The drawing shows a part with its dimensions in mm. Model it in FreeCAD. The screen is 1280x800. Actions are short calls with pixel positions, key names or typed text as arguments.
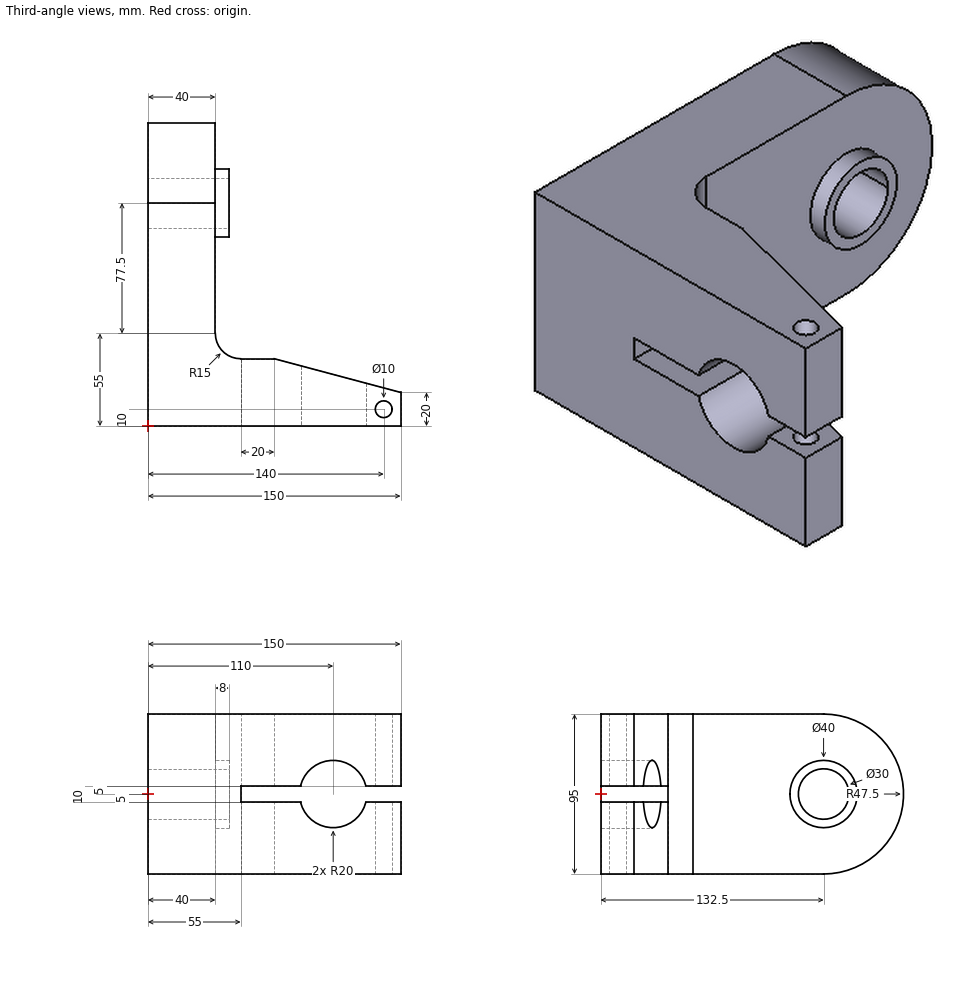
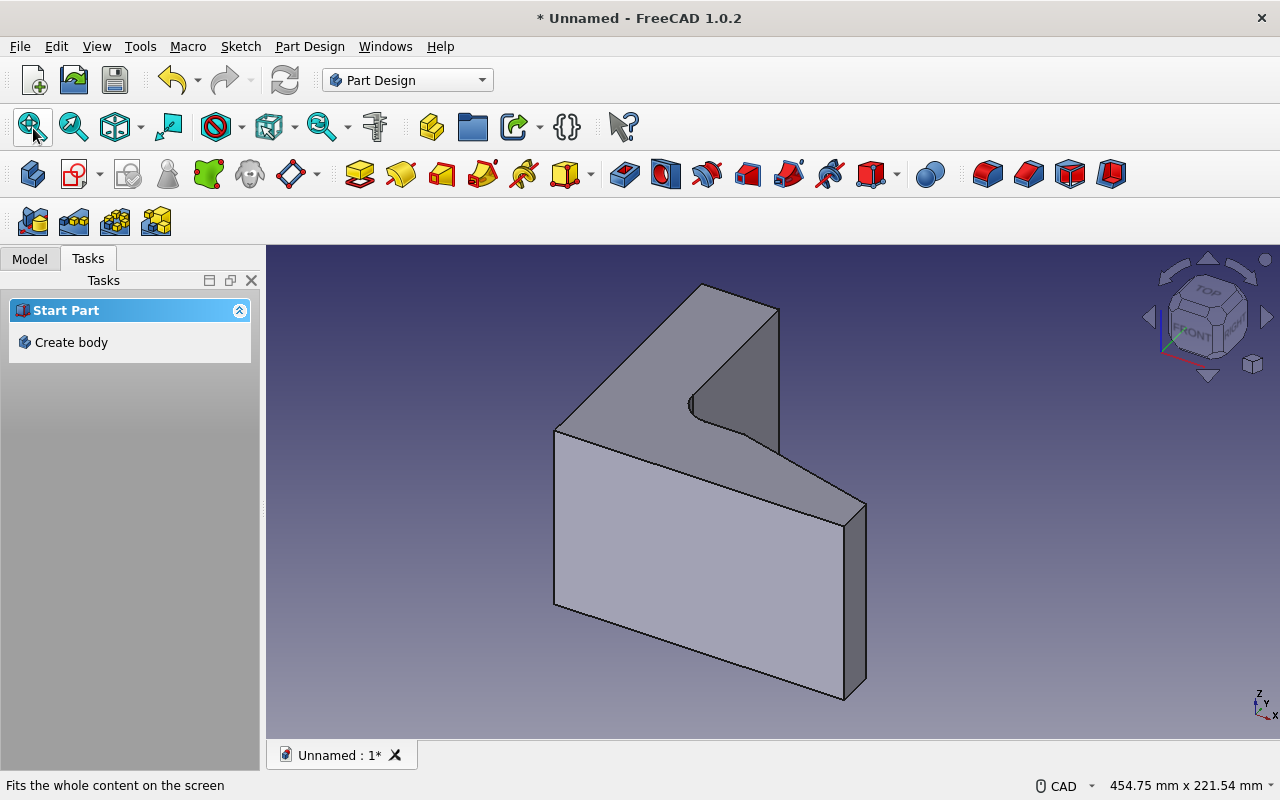
click(74, 174)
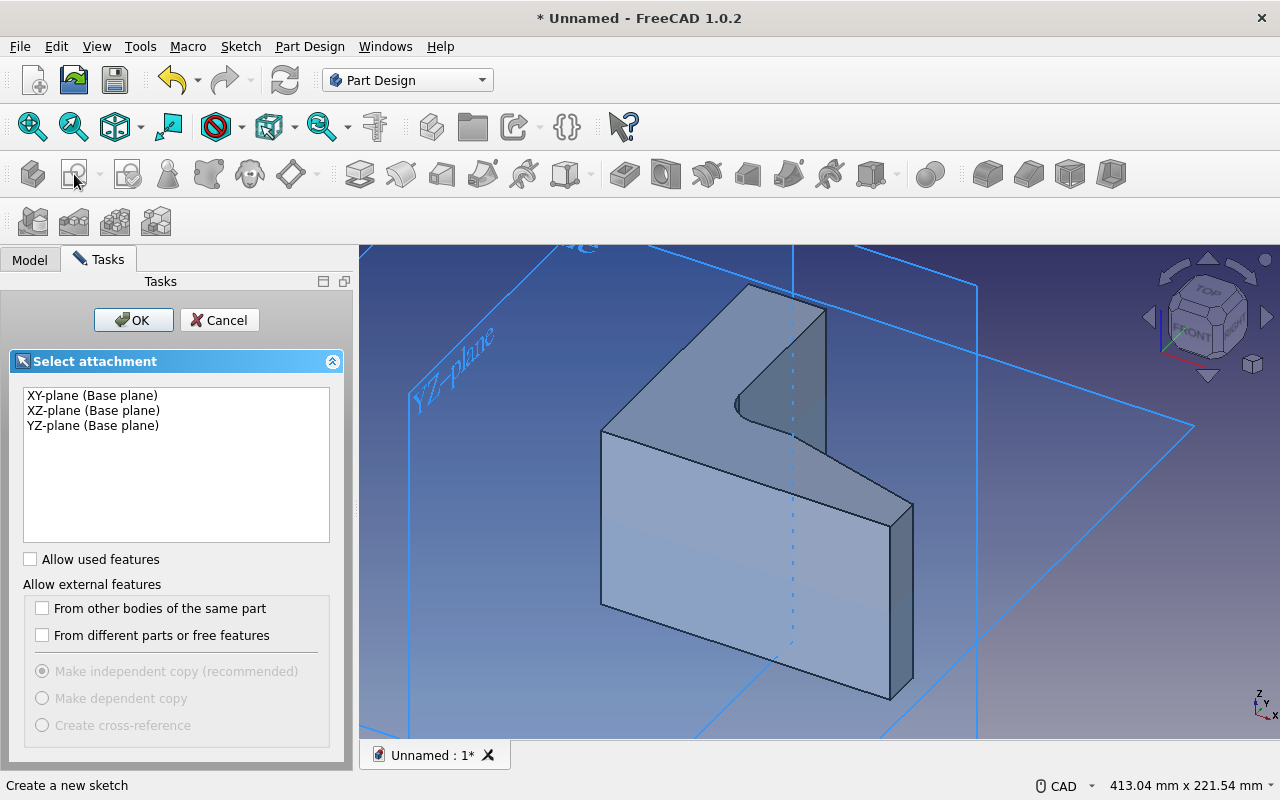
click(84, 426)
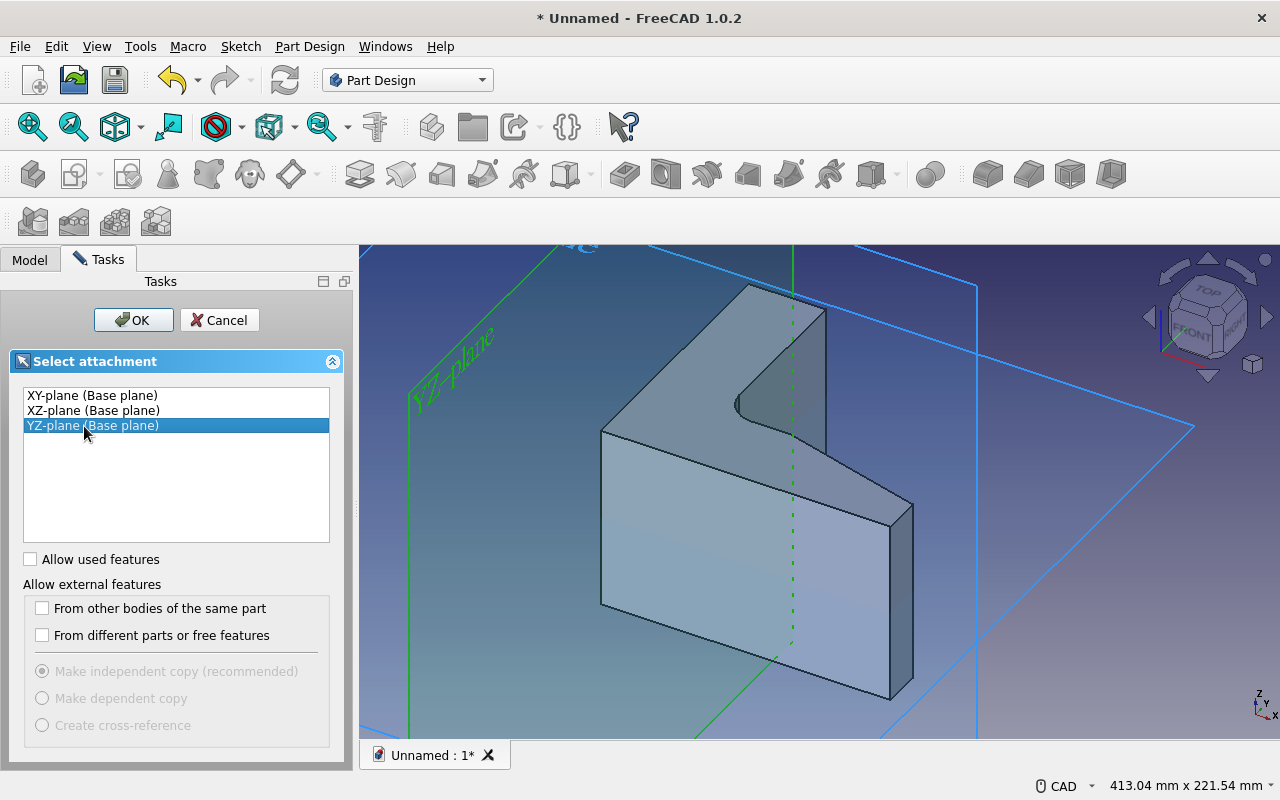
click(134, 320)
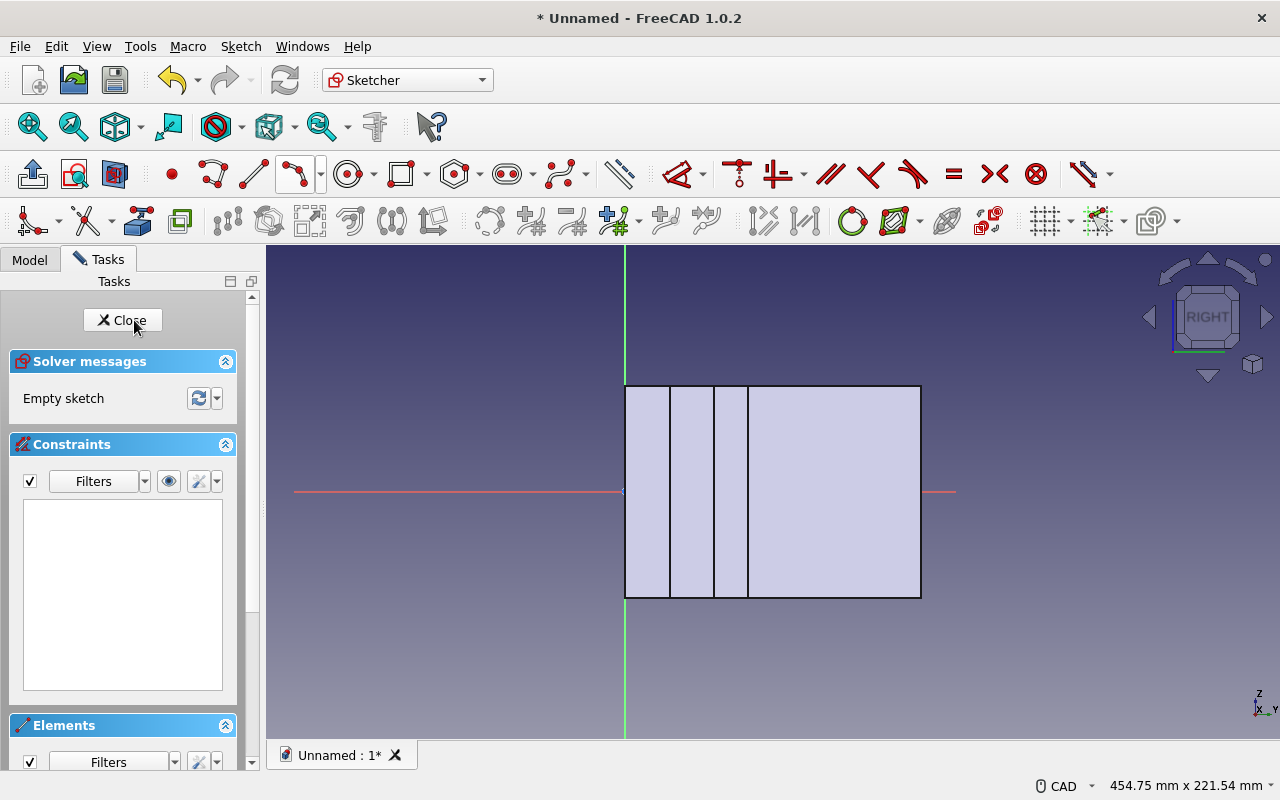
click(115, 174)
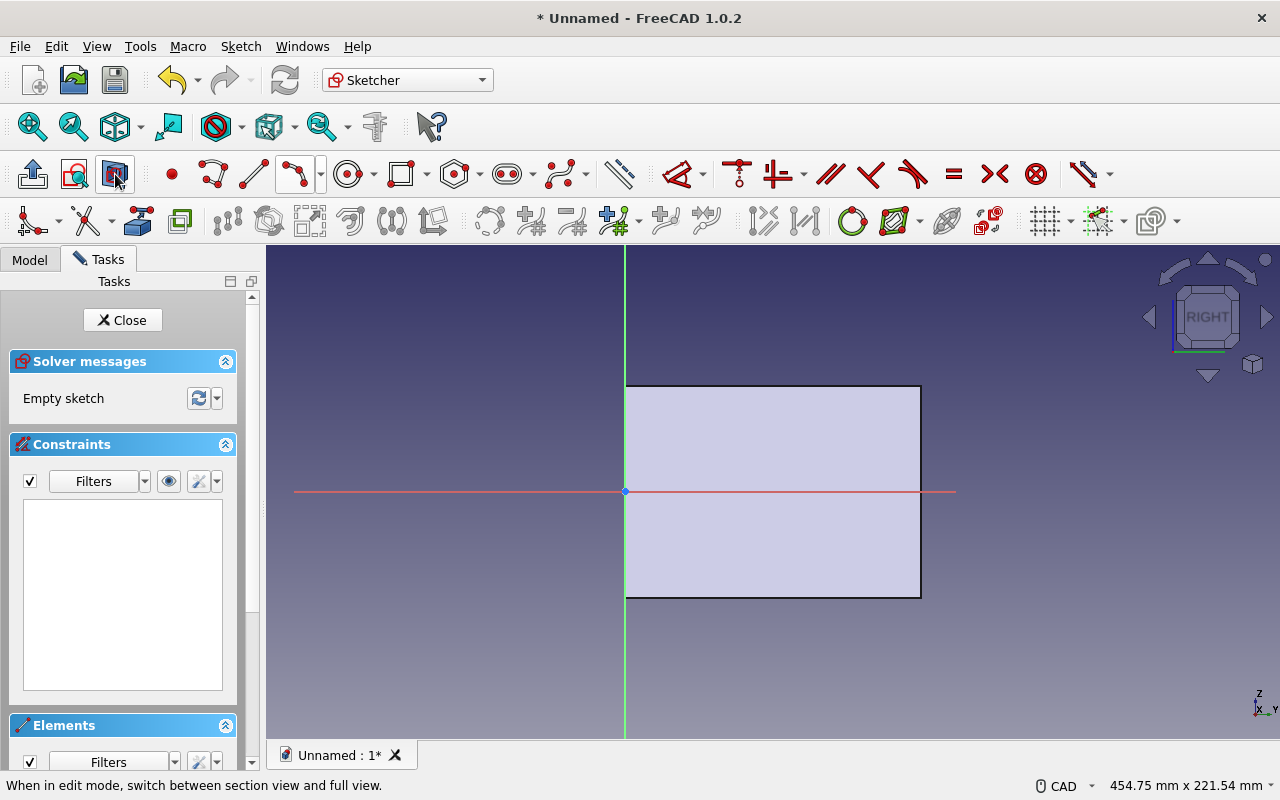
scroll(1073, 492, up, 2)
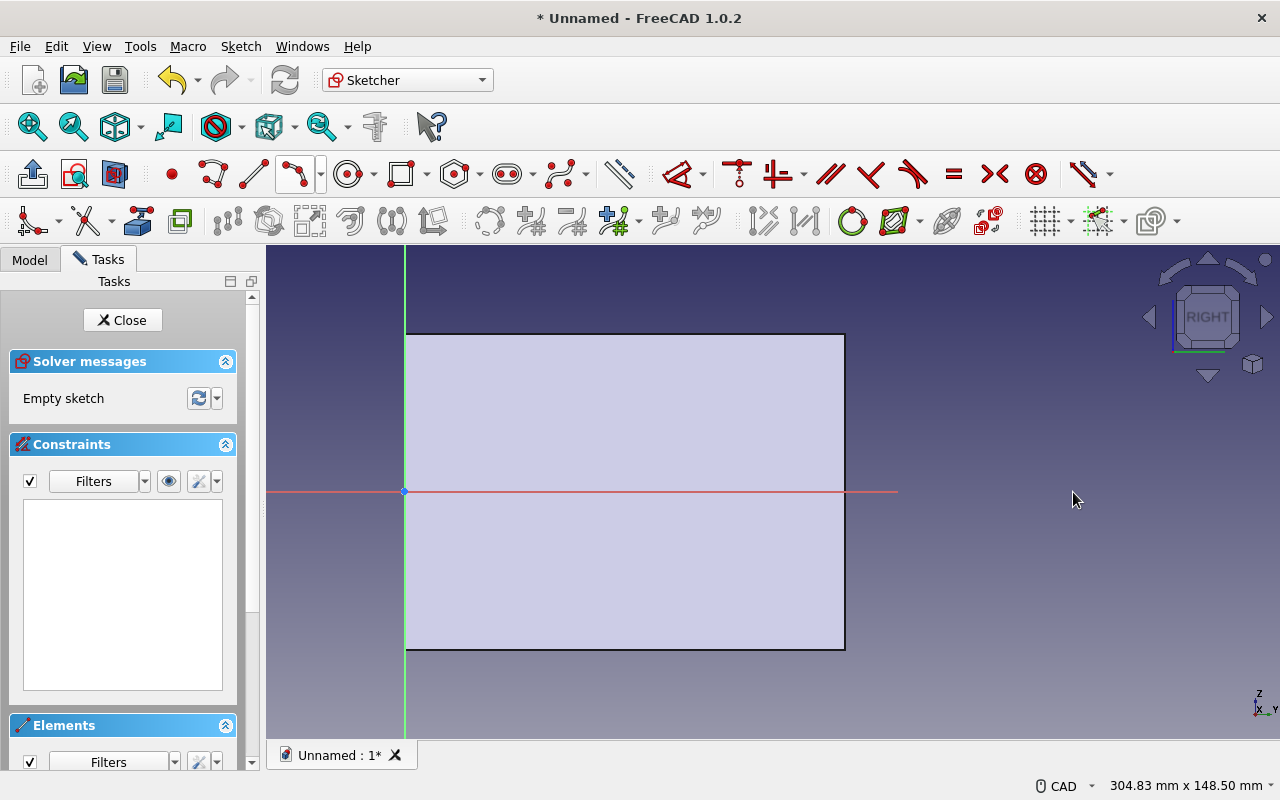
click(254, 174)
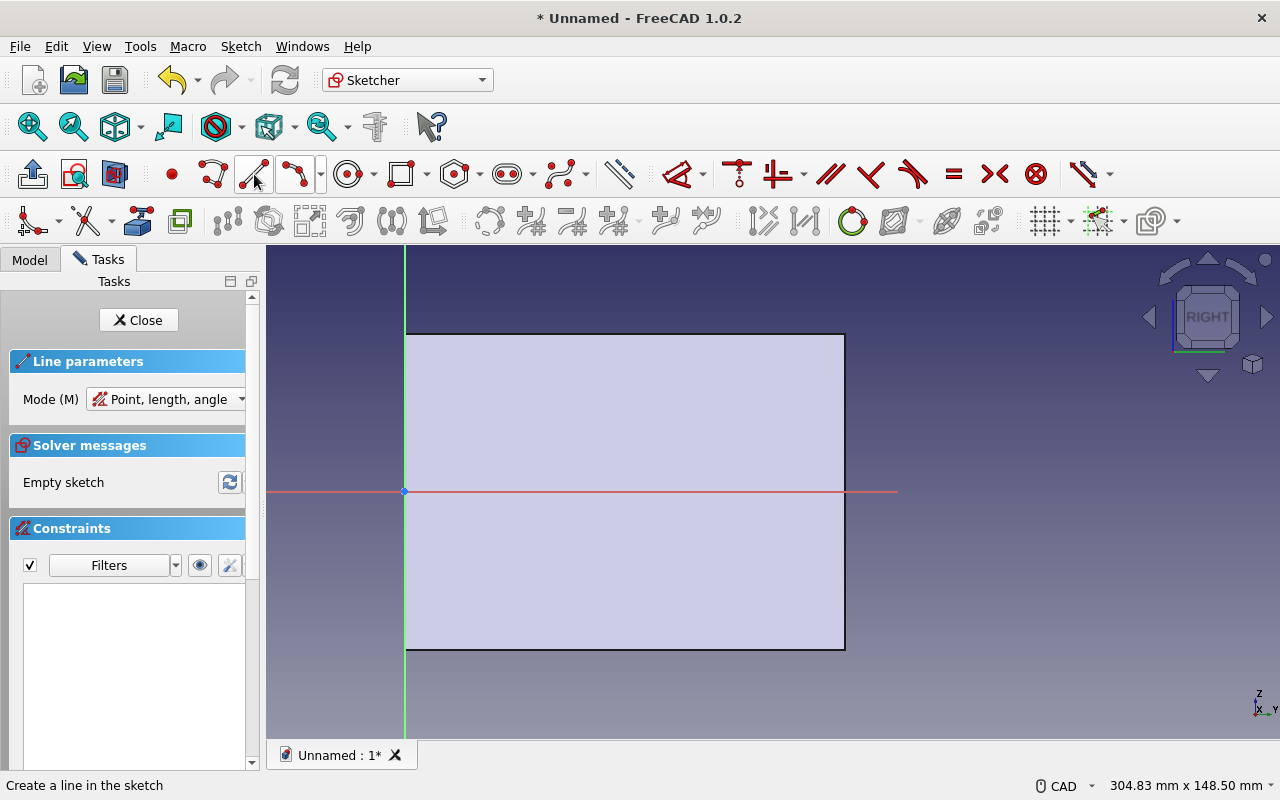
click(845, 650)
click(845, 334)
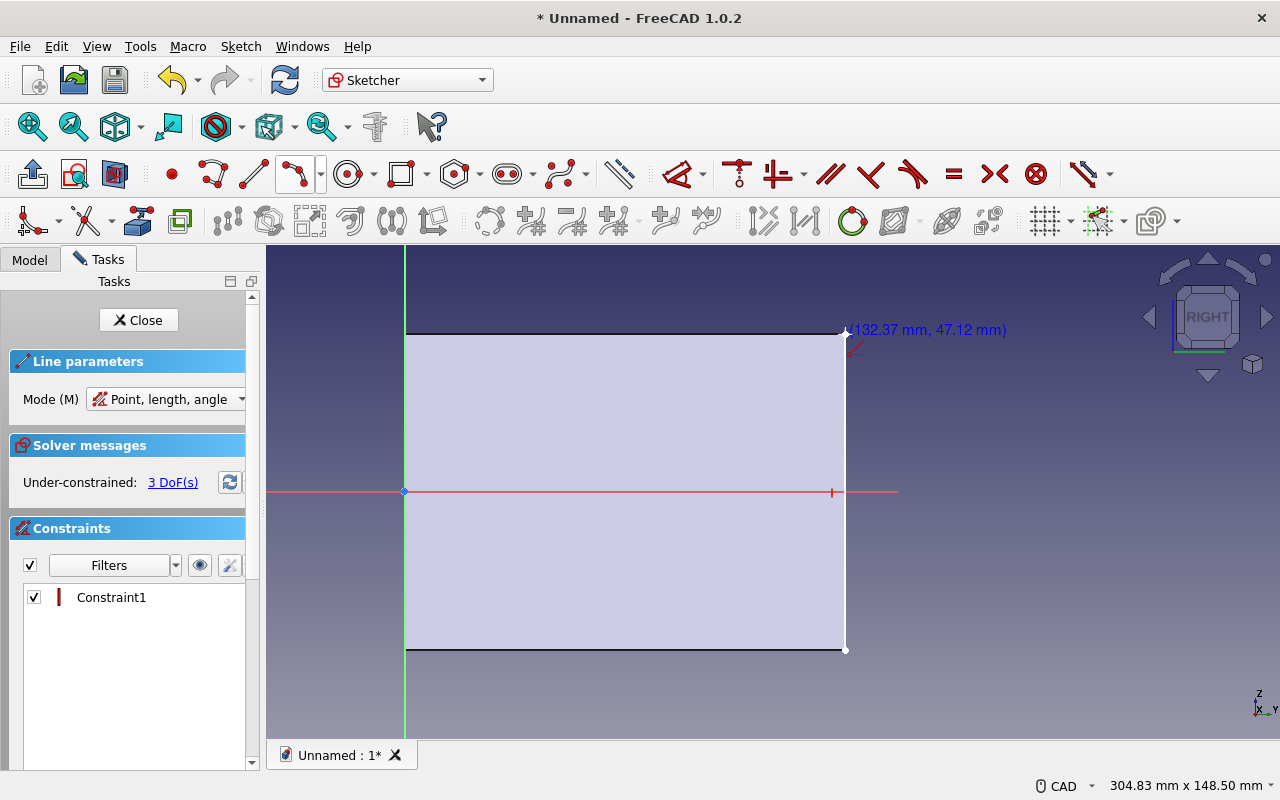
click(294, 174)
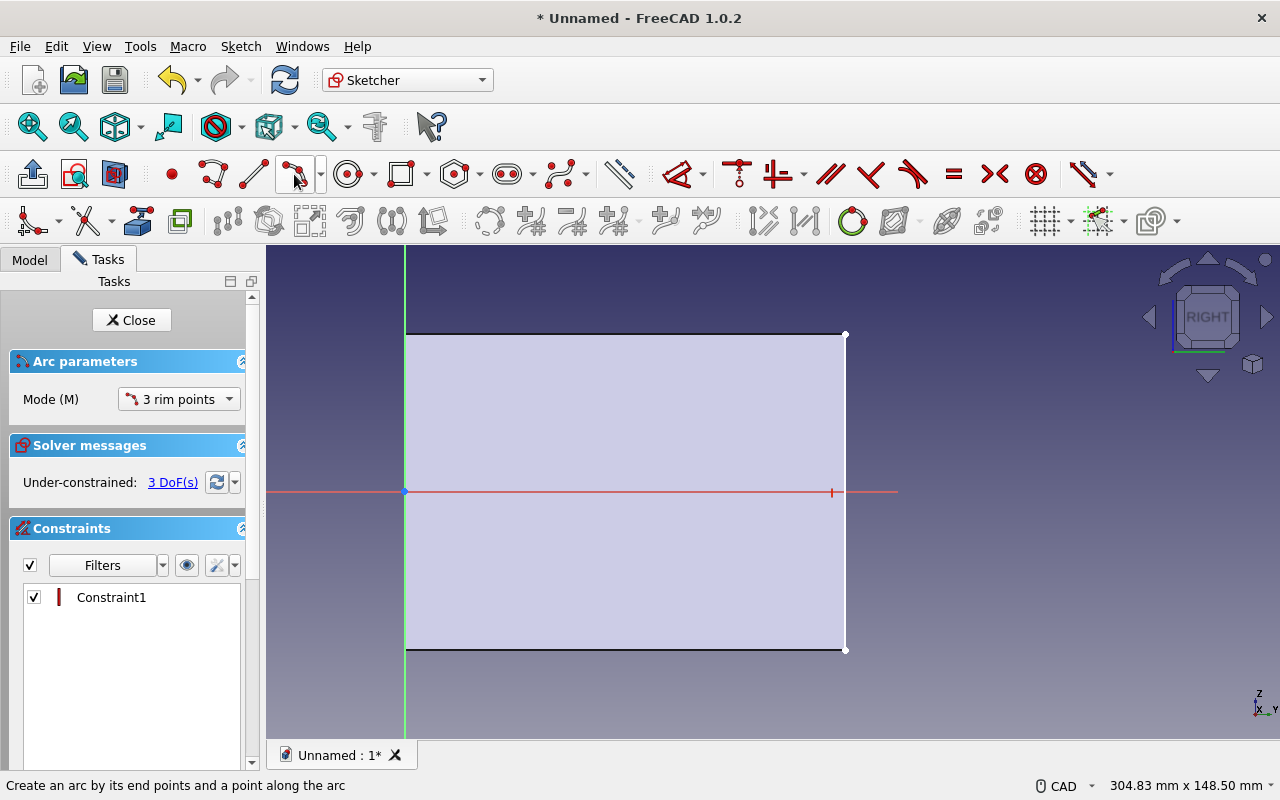
click(845, 335)
click(845, 651)
click(996, 541)
key(Escape)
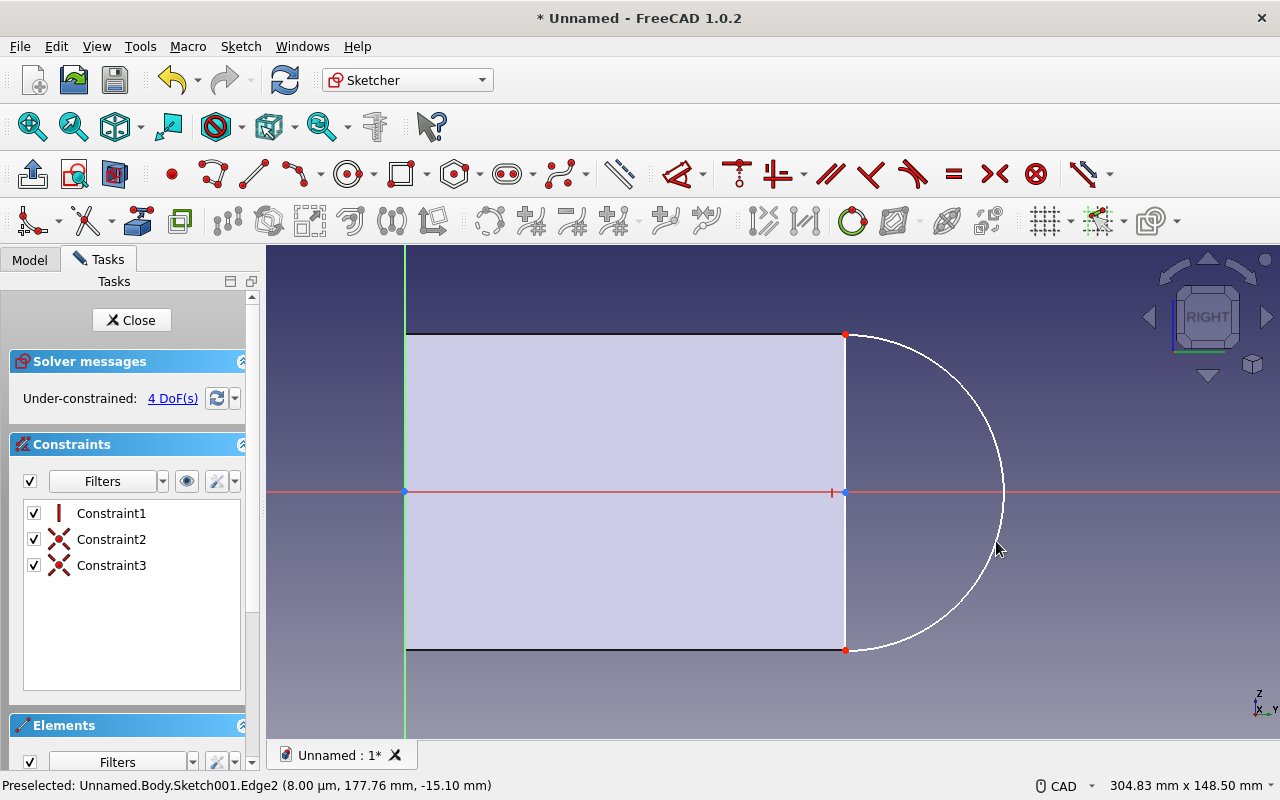
click(846, 493)